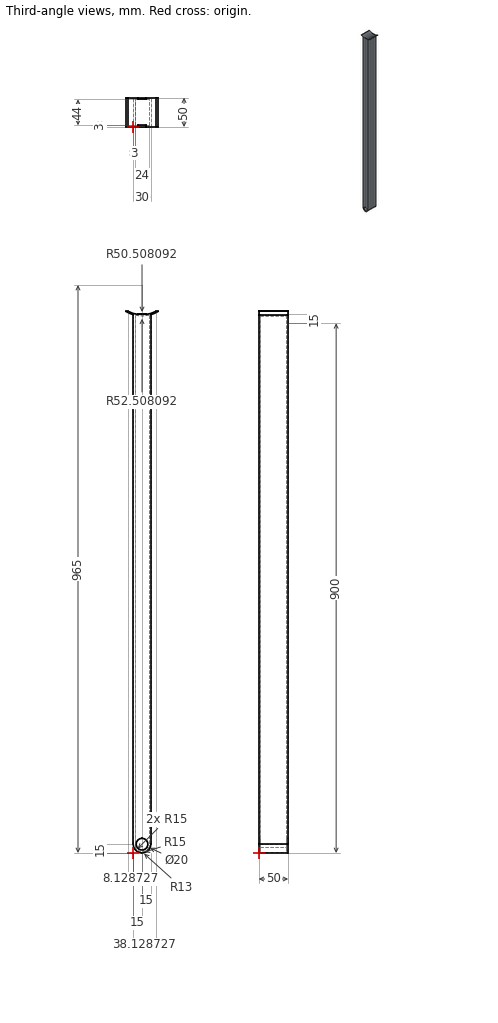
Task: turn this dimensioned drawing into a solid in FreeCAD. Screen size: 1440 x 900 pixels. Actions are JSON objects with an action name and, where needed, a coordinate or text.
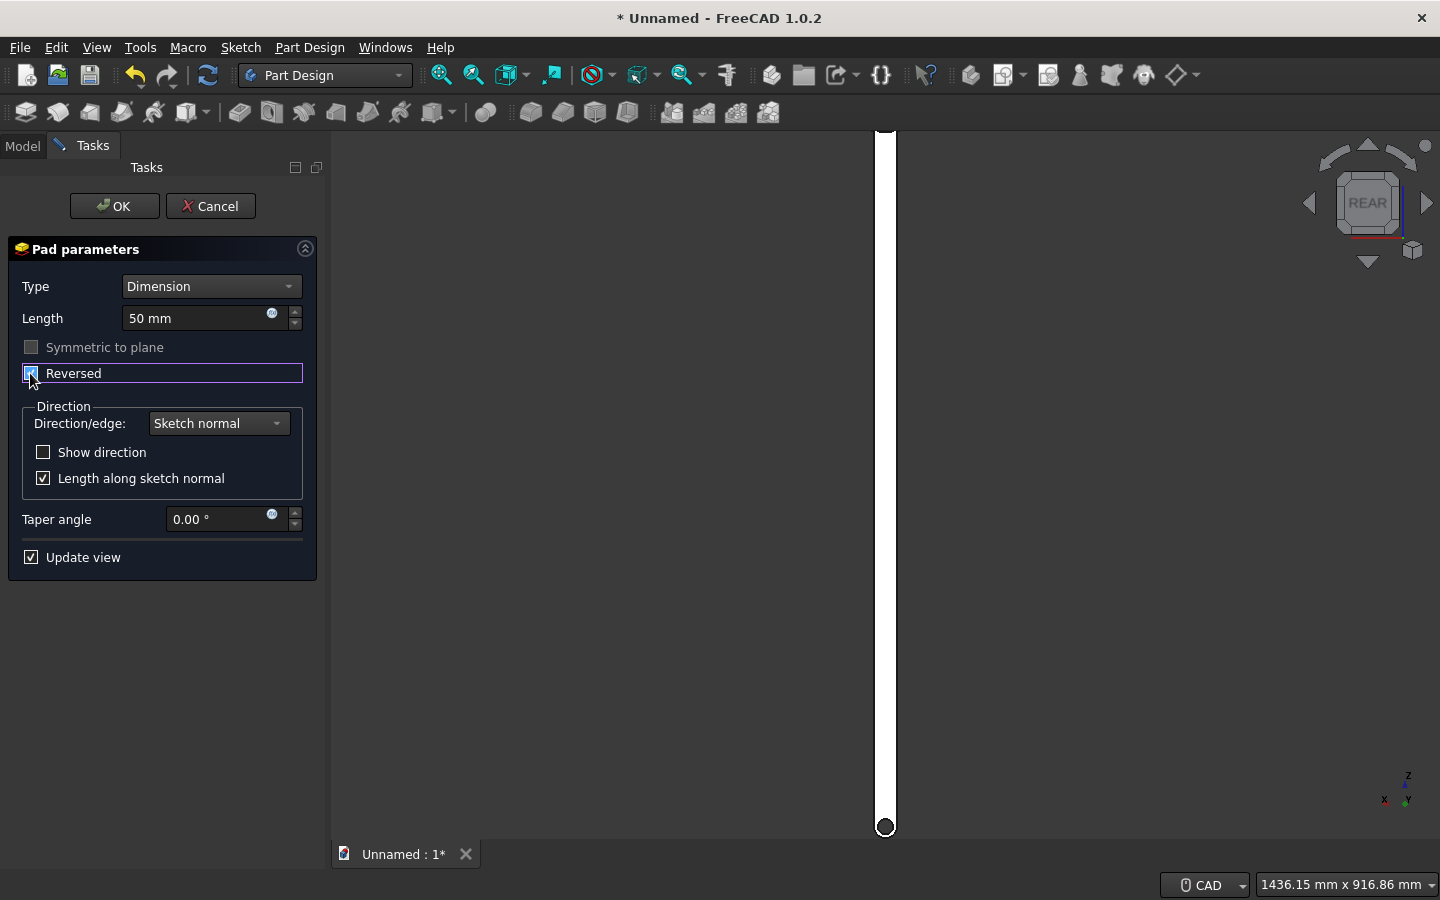
{"action": "left_click", "coordinate": [115, 206]}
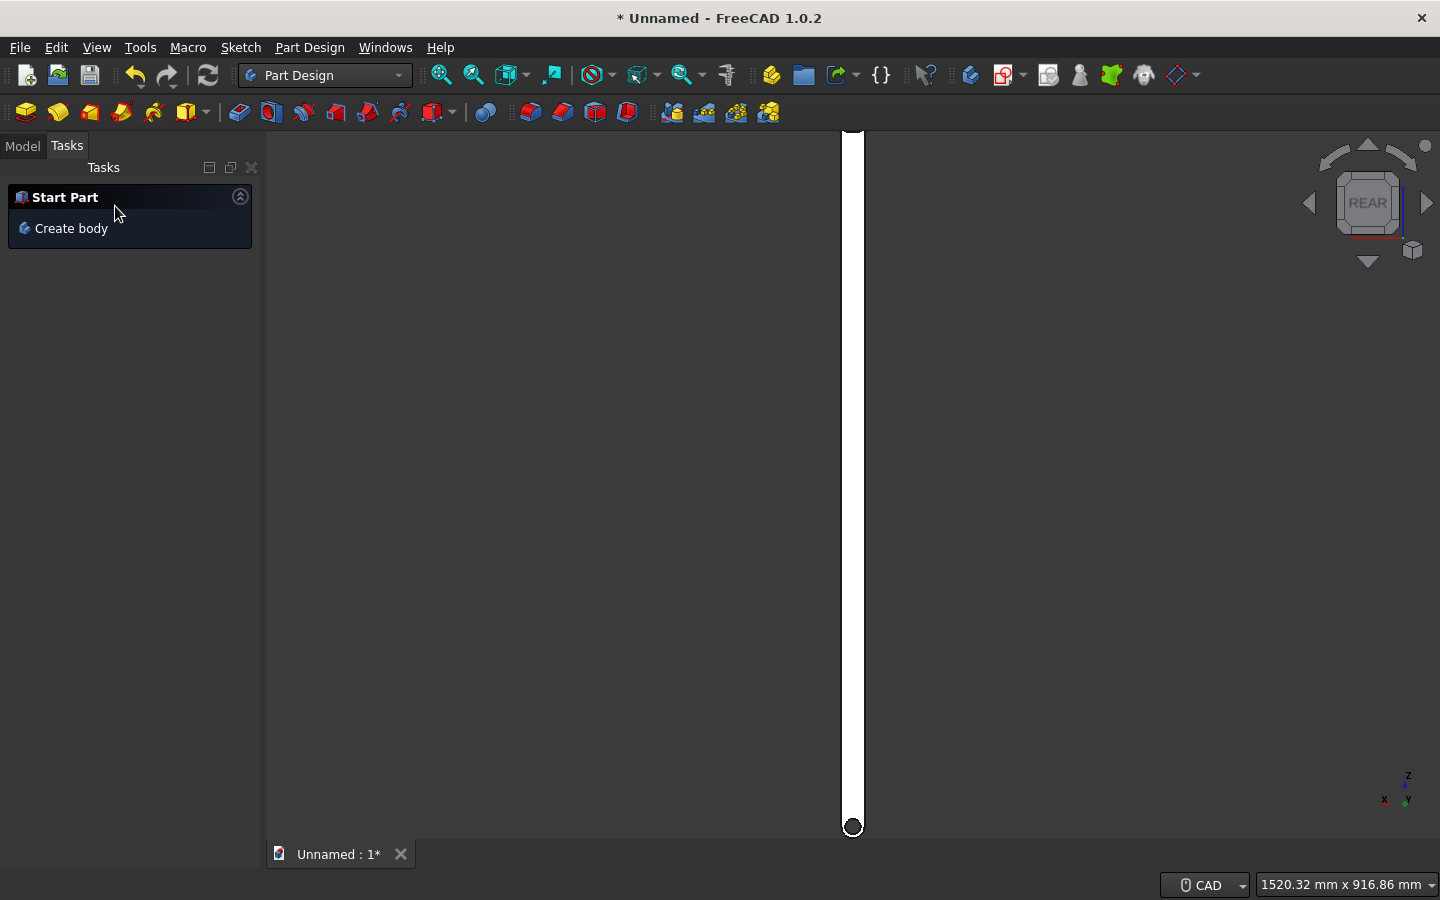
{"action": "key", "text": "0"}